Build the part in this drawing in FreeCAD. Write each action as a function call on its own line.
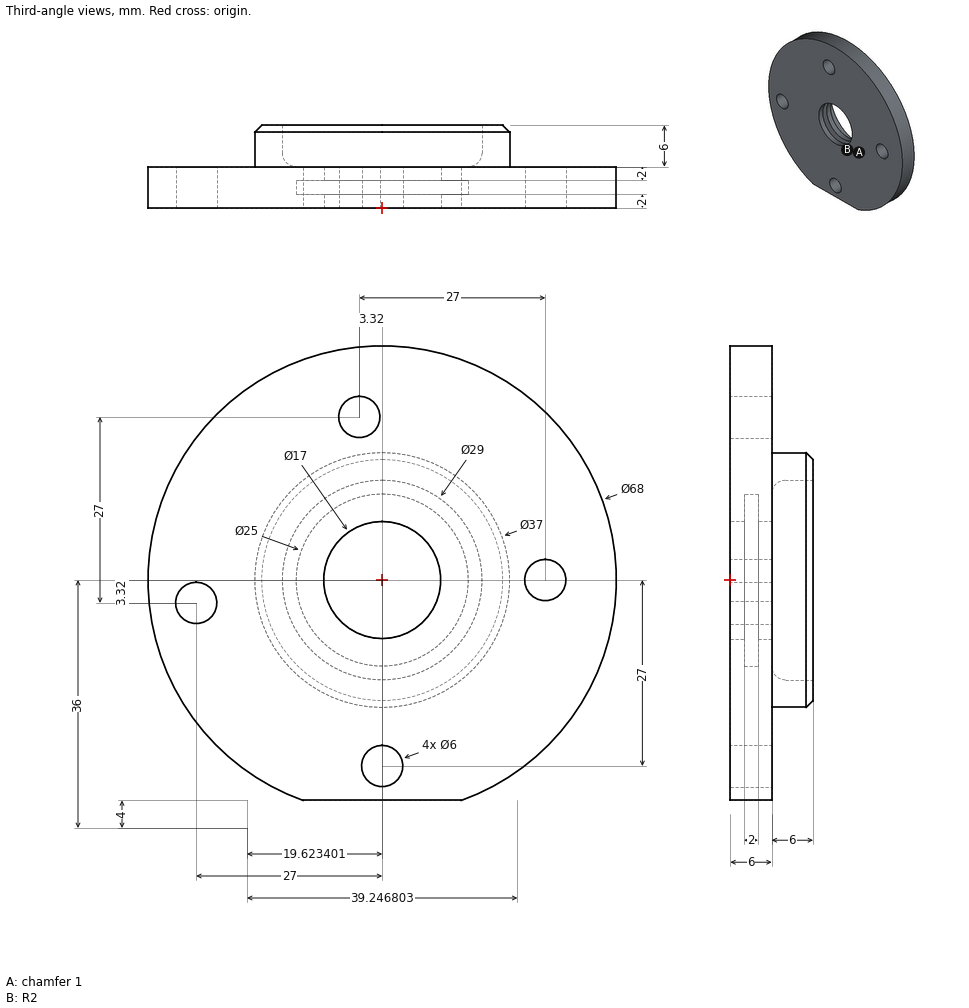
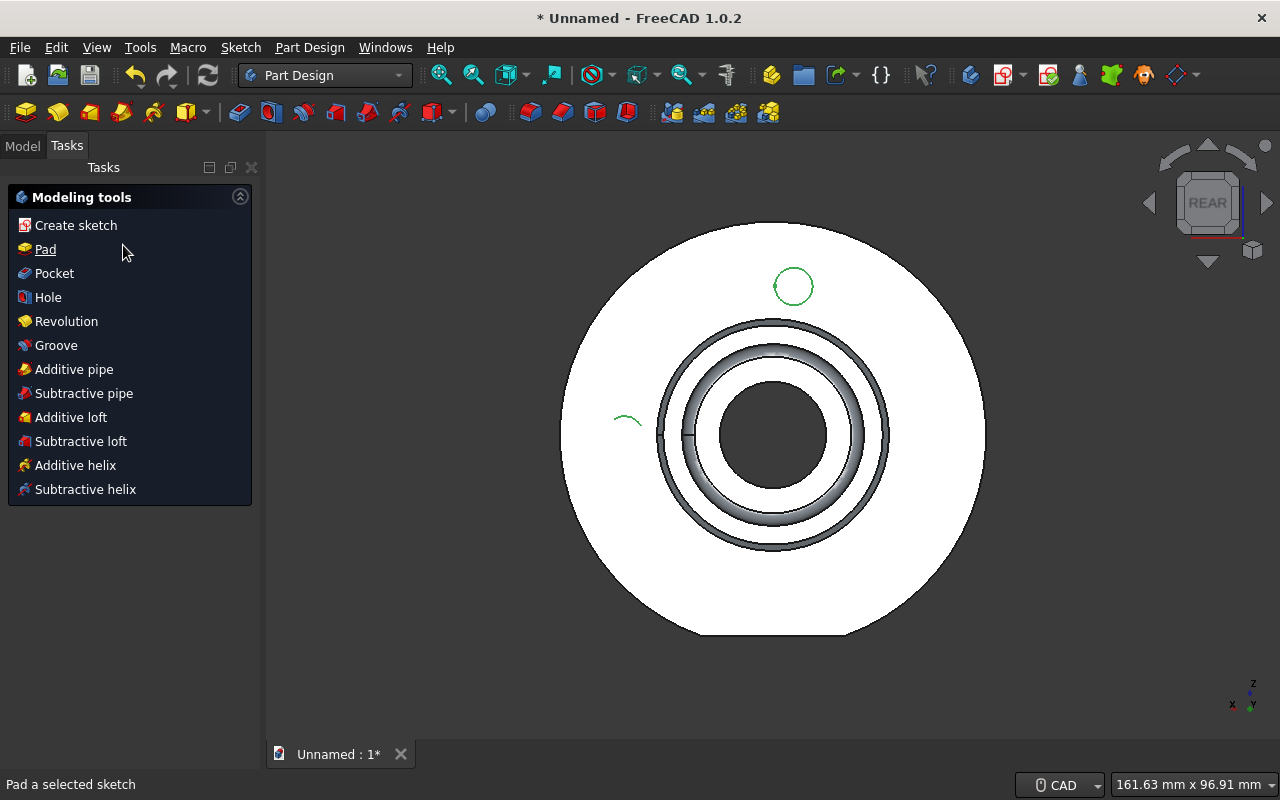
click(240, 112)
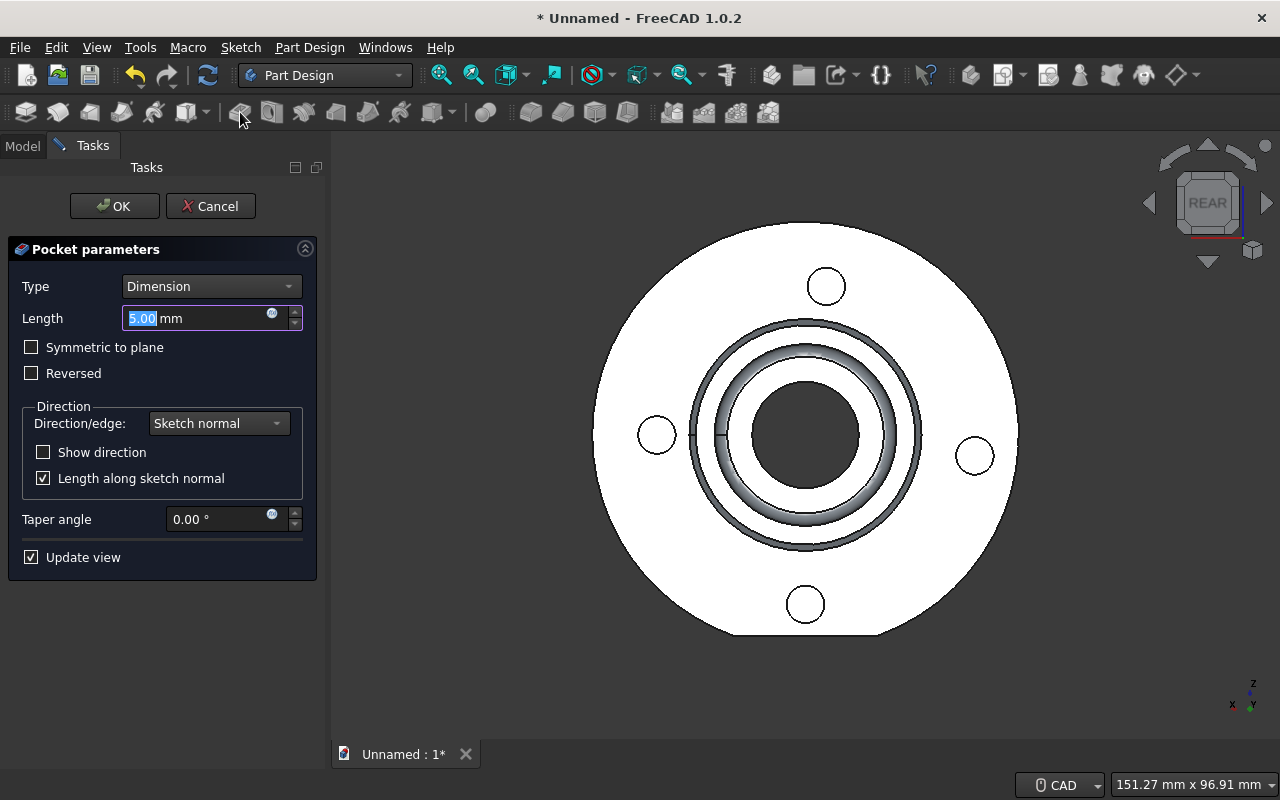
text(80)
key(Tab)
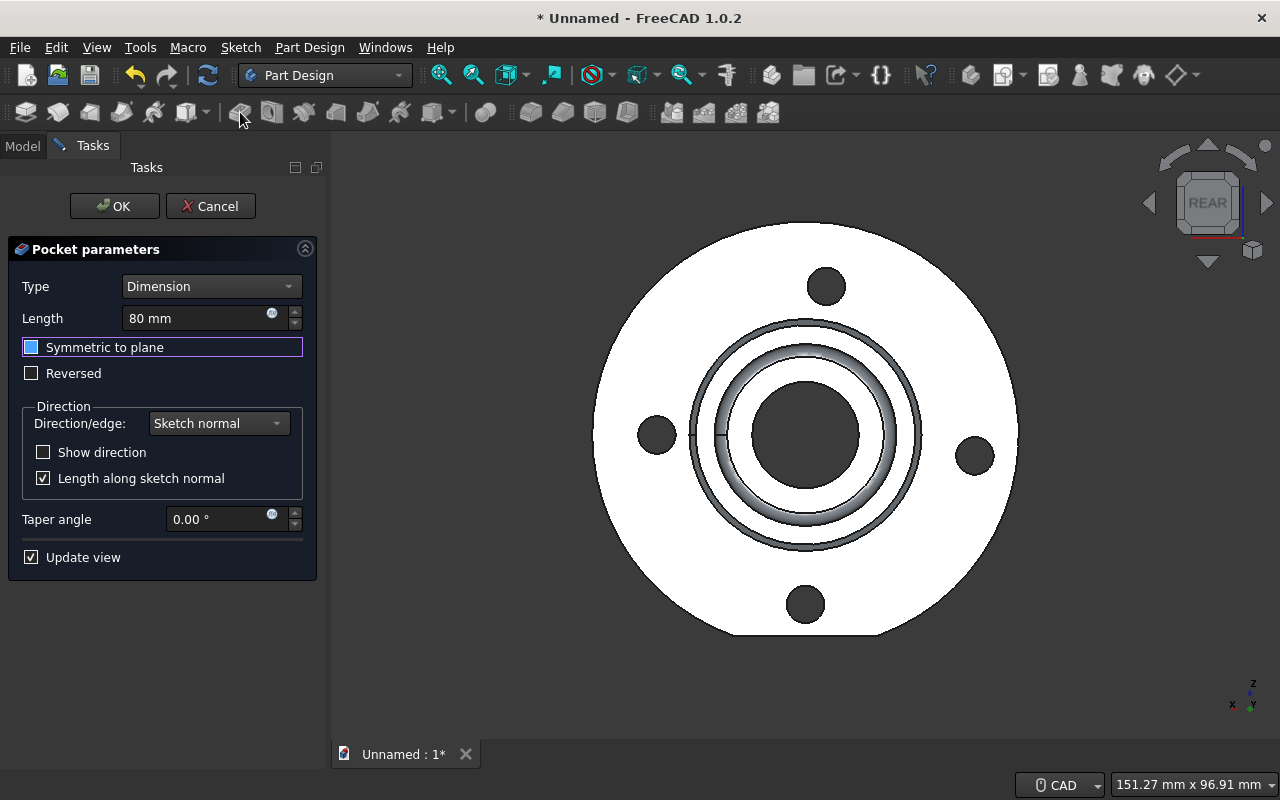
click(115, 206)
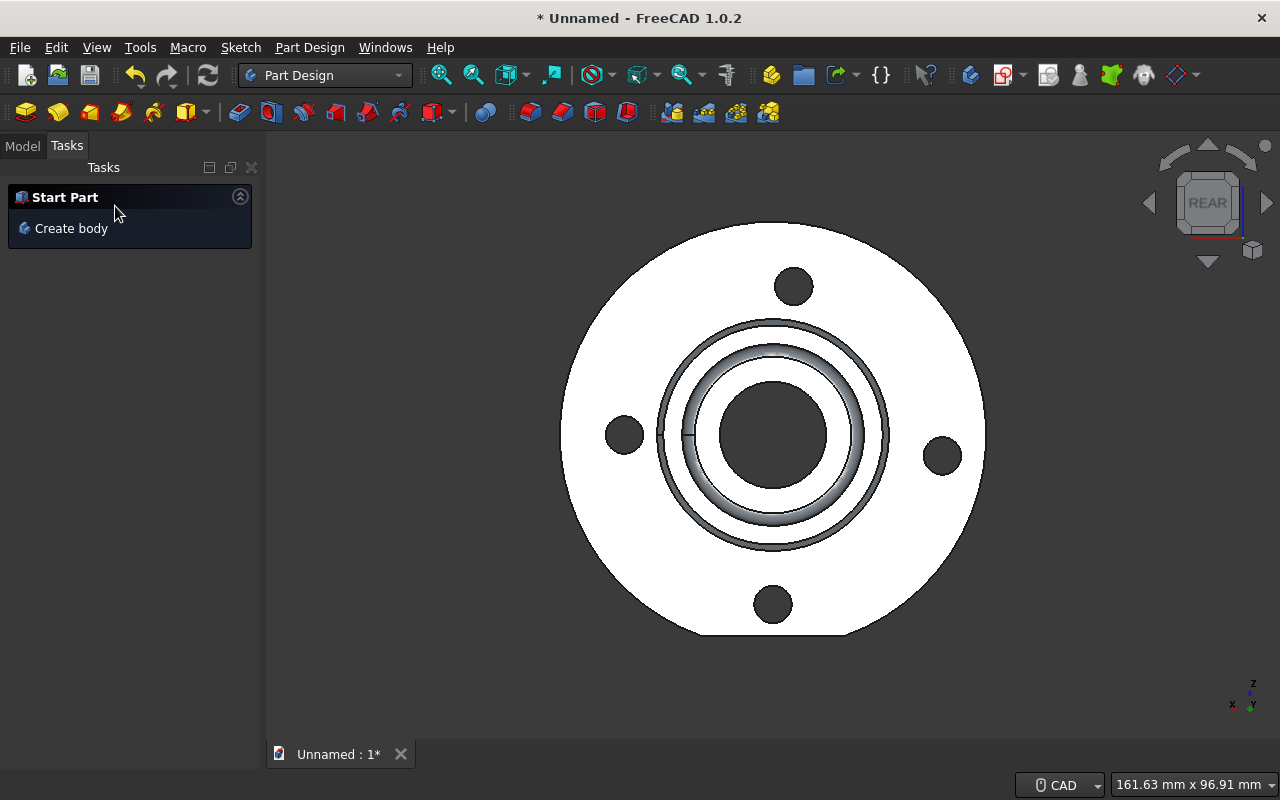
key(0)